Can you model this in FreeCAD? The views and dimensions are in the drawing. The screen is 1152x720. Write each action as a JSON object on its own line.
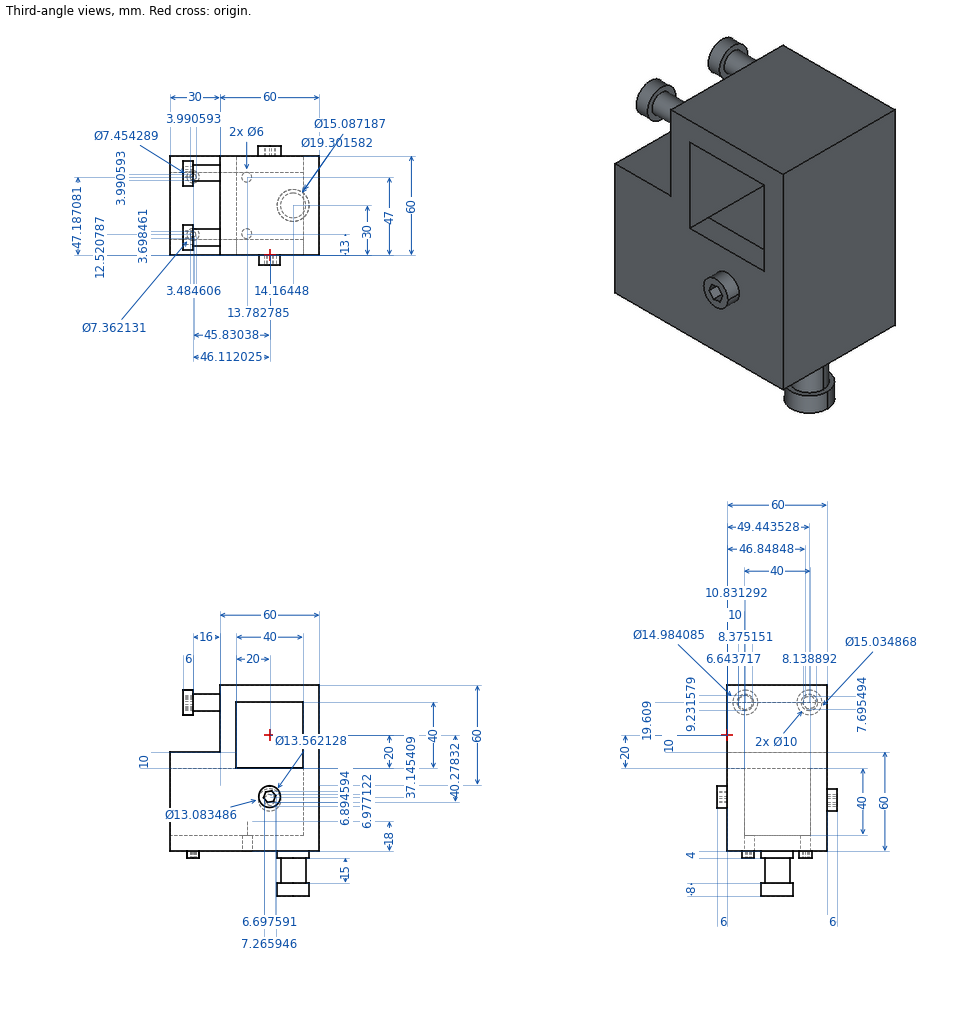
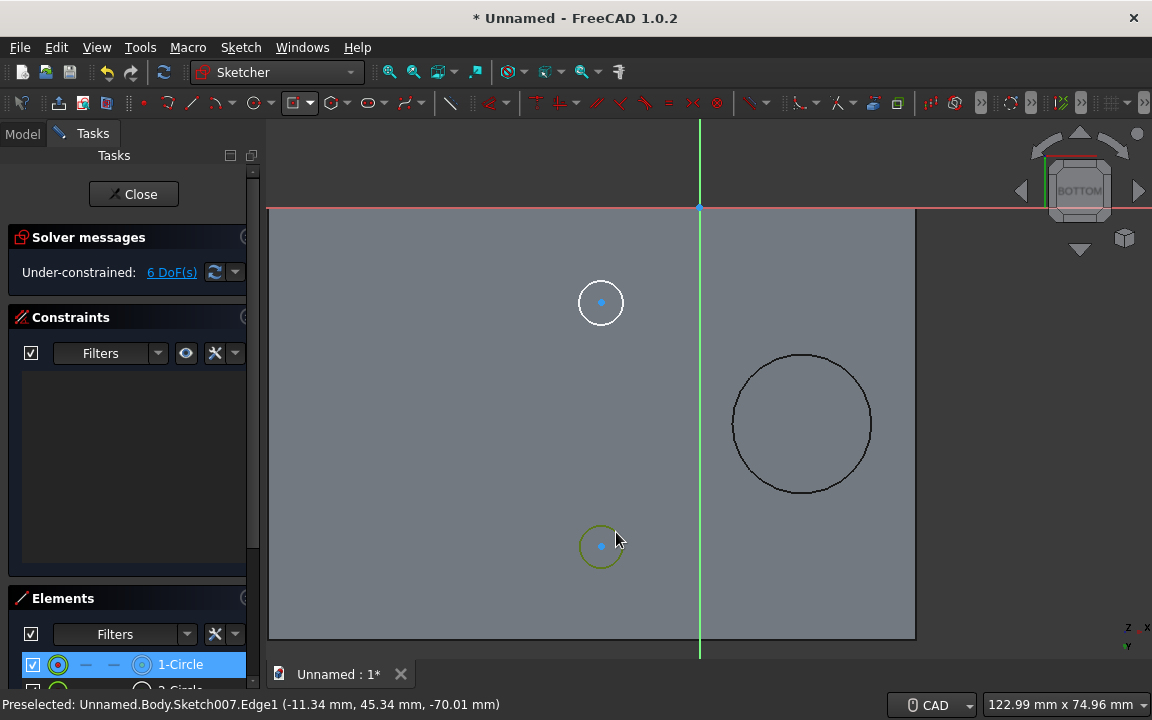
{"action": "left_click", "coordinate": [616, 287]}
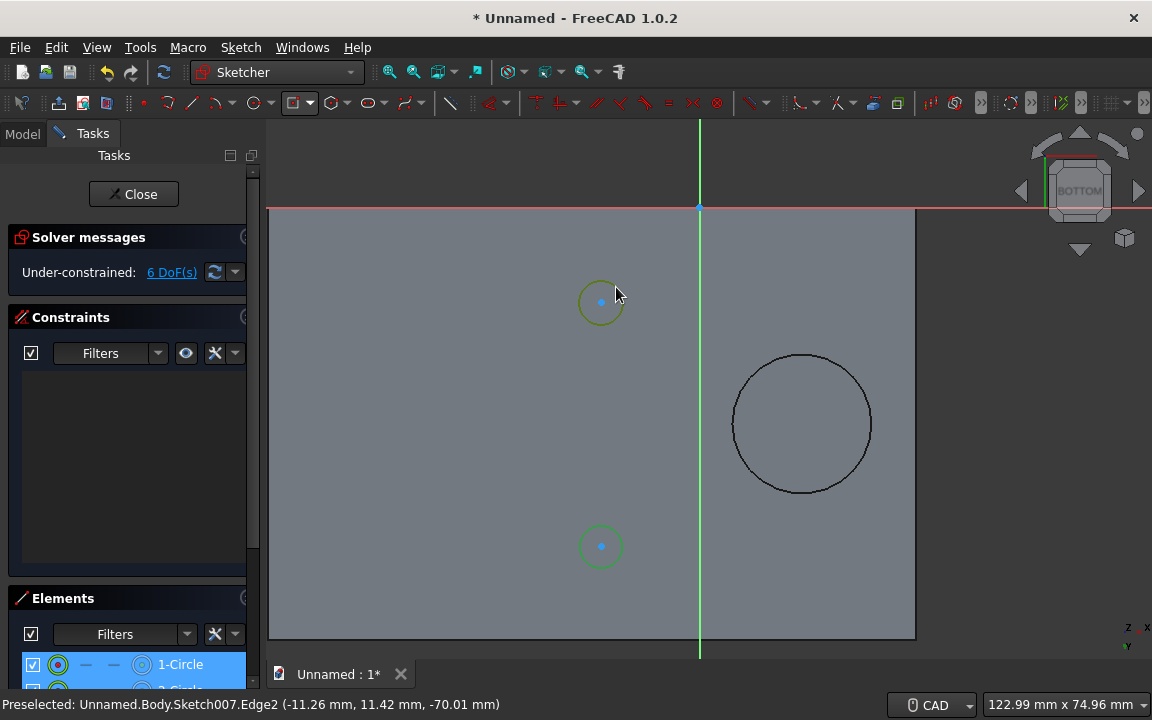
{"action": "left_click", "coordinate": [670, 104]}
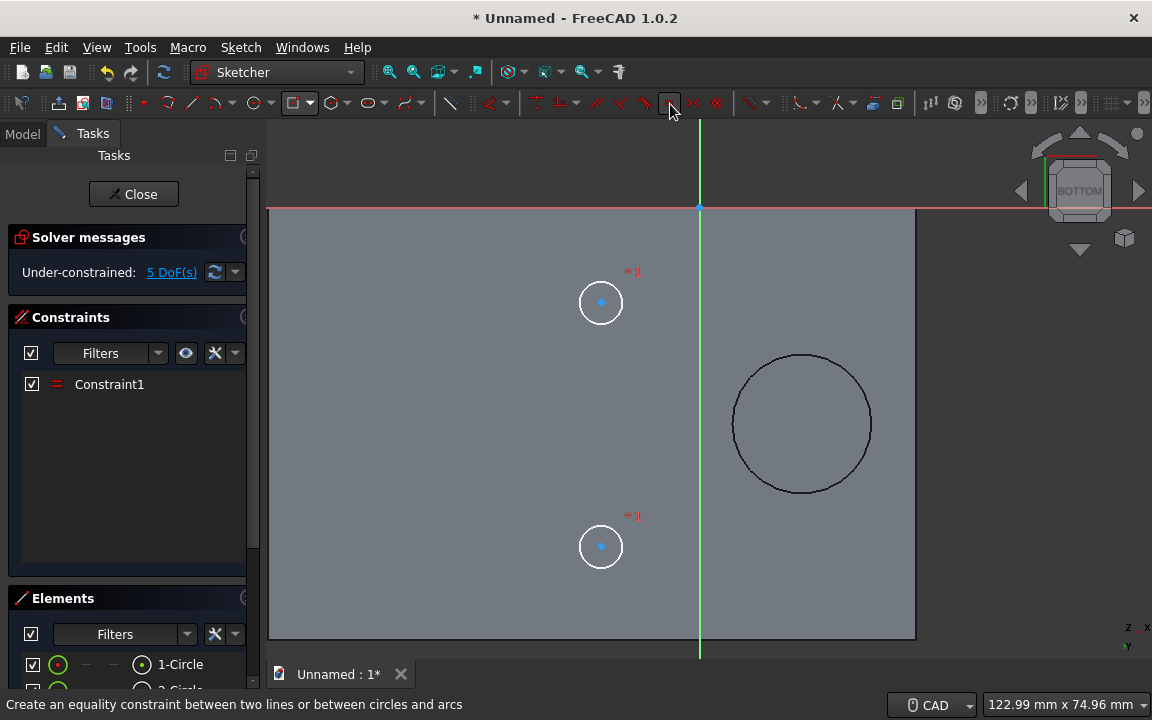
{"action": "left_click", "coordinate": [601, 547]}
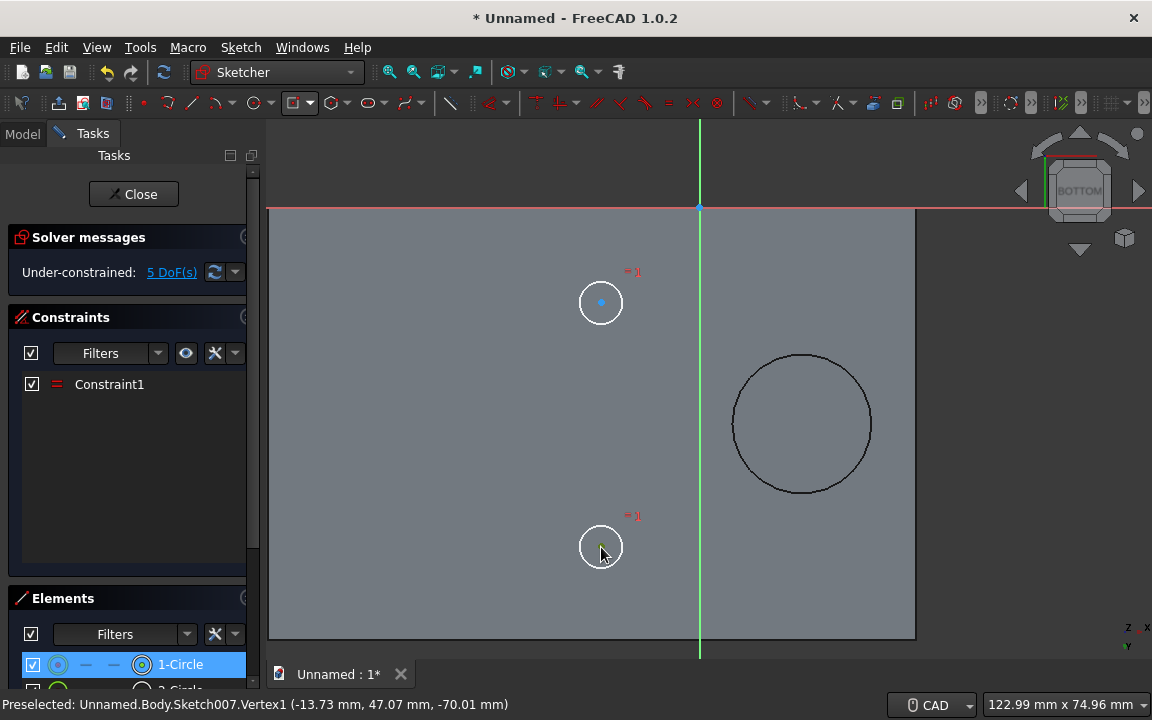
{"action": "left_click", "coordinate": [601, 303]}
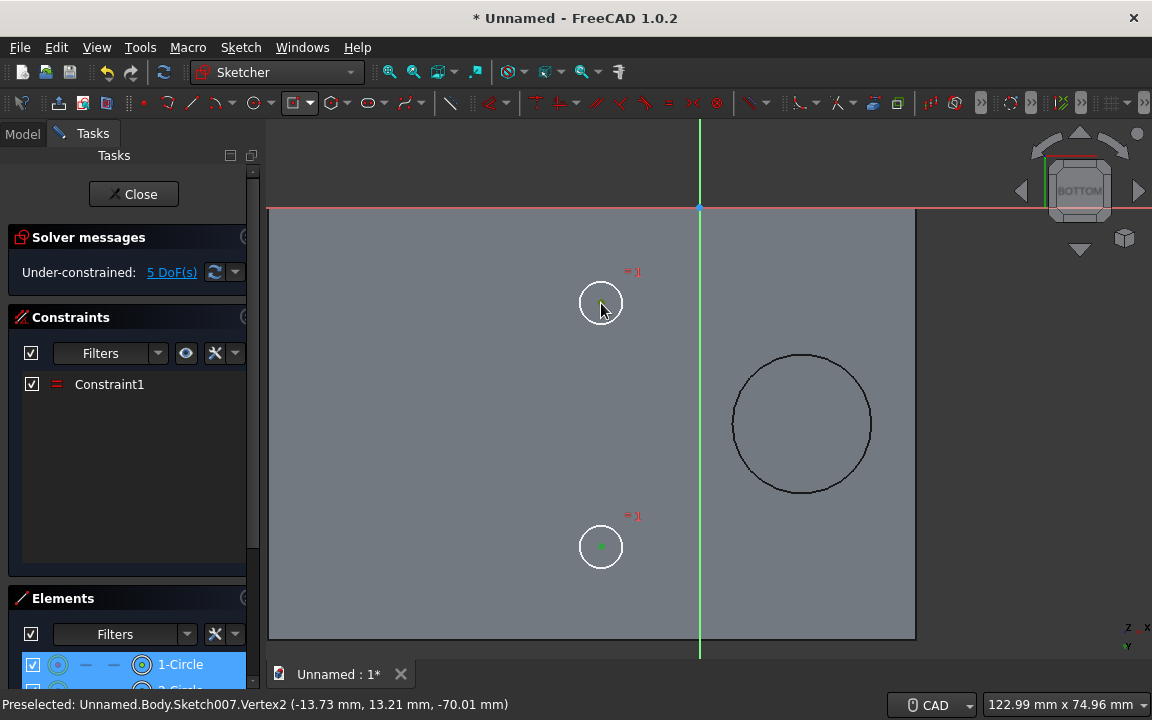
{"action": "left_click", "coordinate": [578, 104]}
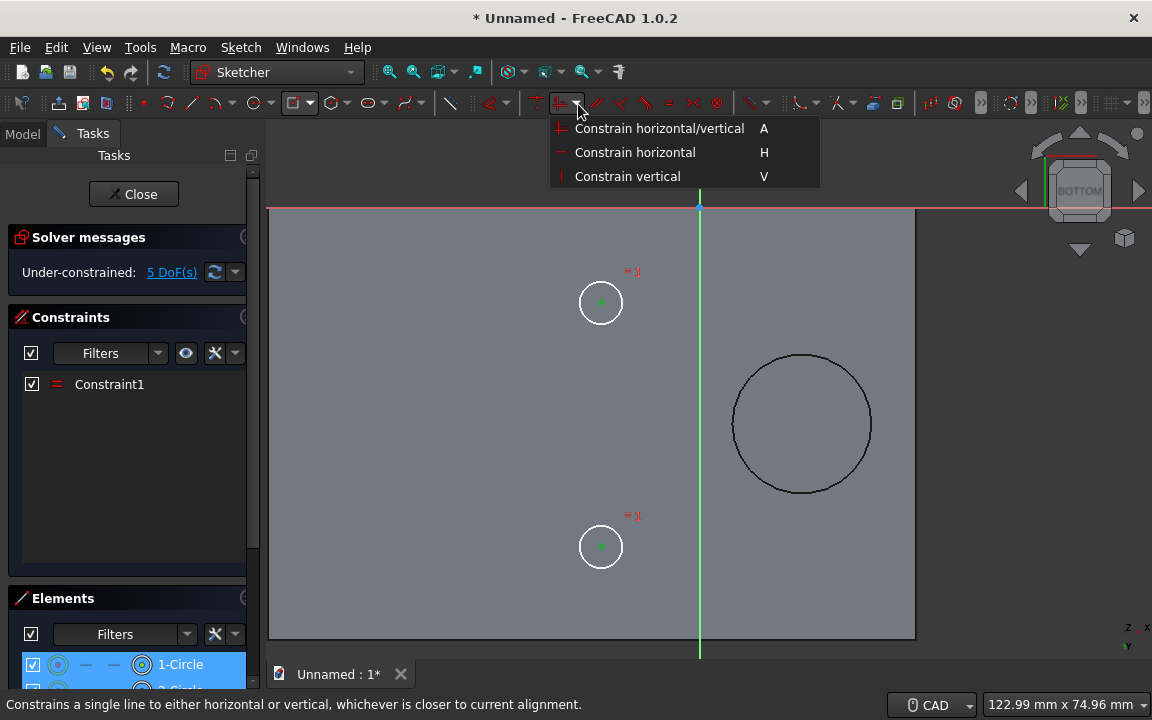
{"action": "left_click", "coordinate": [685, 176]}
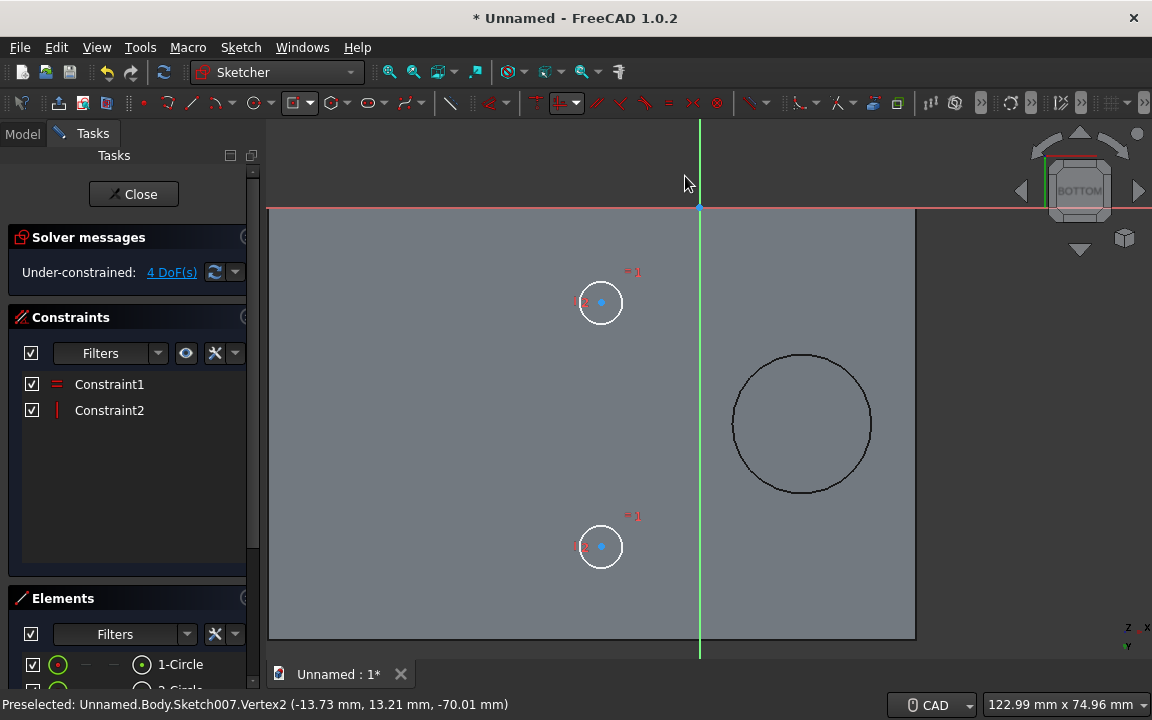
{"action": "left_click", "coordinate": [490, 104]}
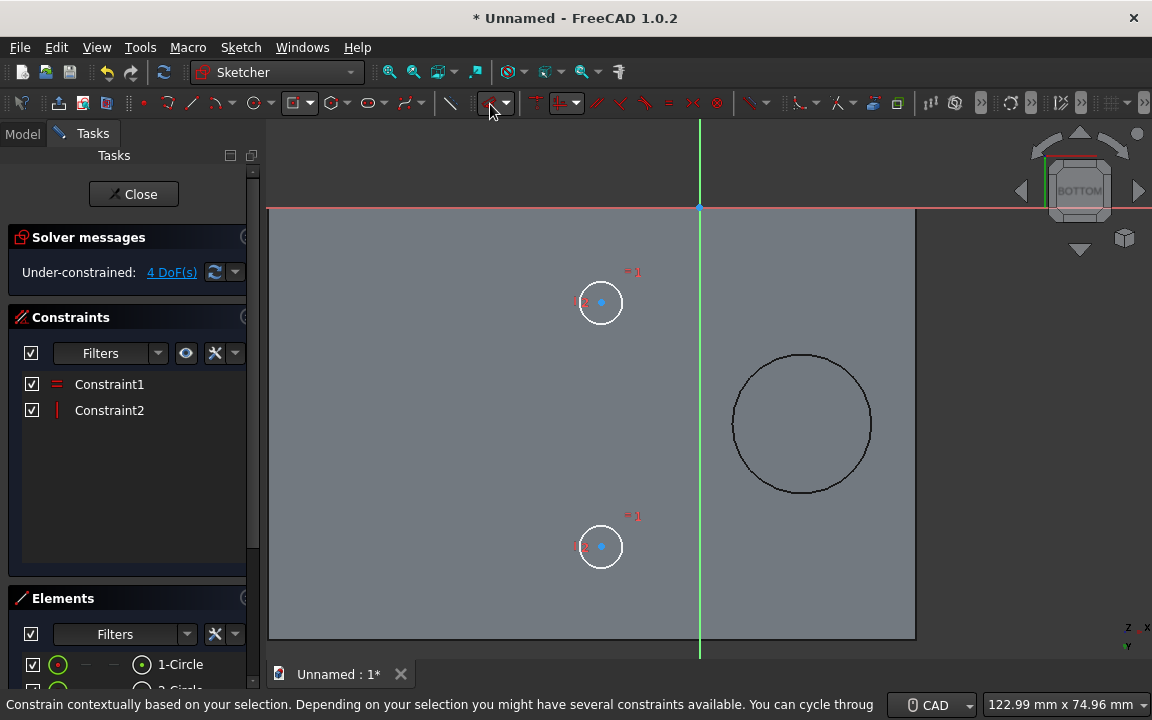
{"action": "left_click", "coordinate": [616, 532]}
{"action": "left_click", "coordinate": [639, 509]}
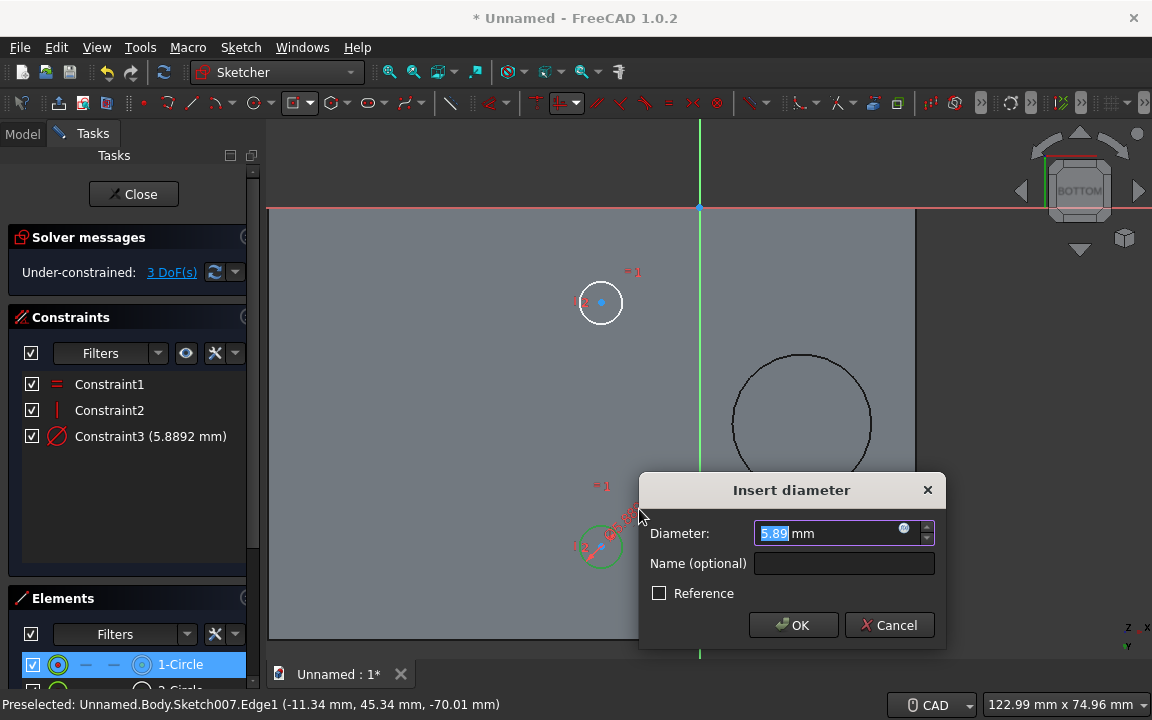
{"action": "type", "text": "6"}
{"action": "key", "text": "Return"}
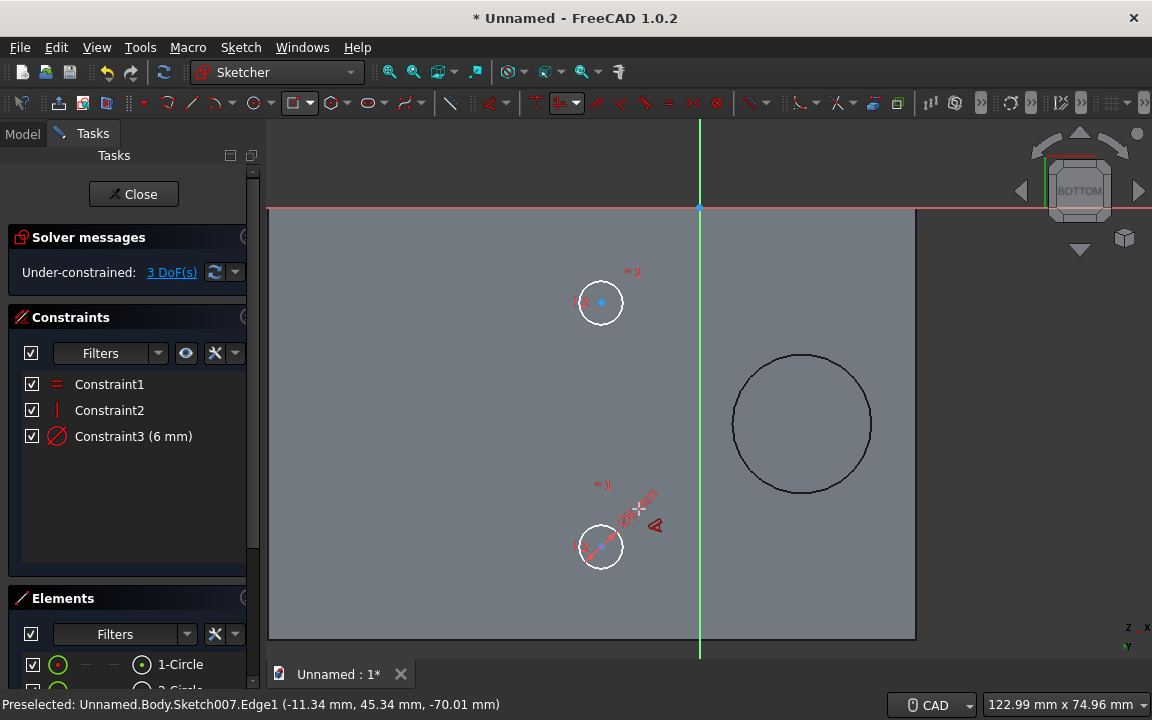
{"action": "left_click", "coordinate": [601, 547]}
{"action": "left_click", "coordinate": [734, 377]}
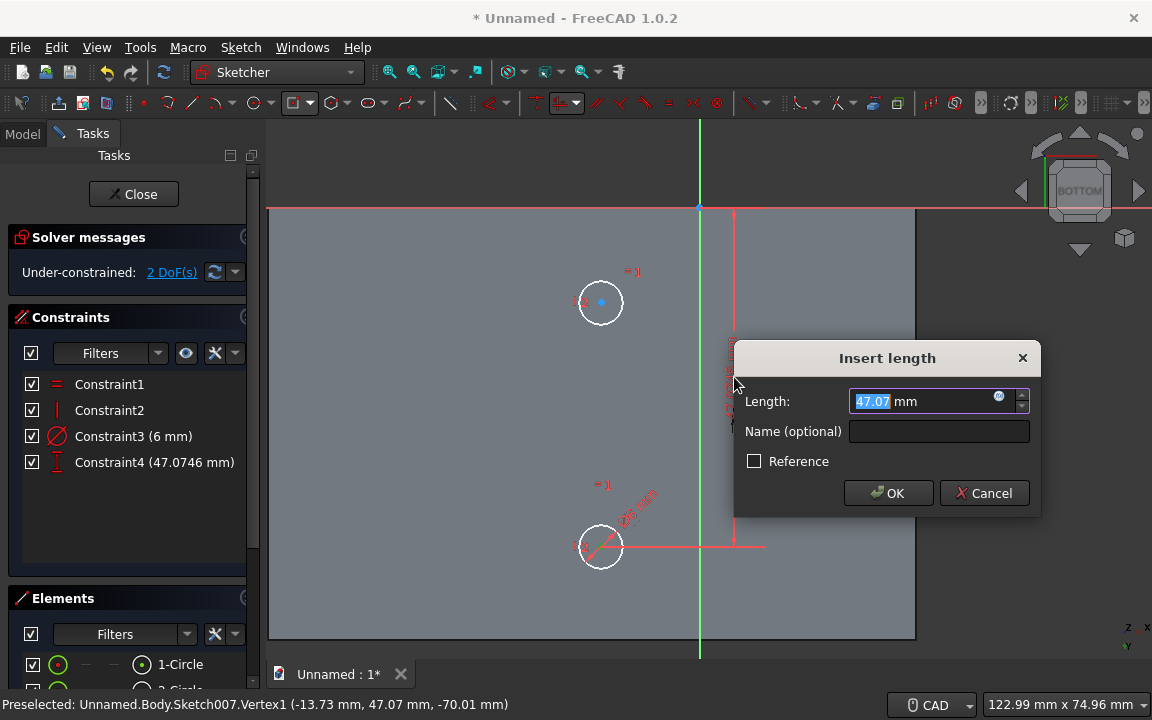
{"action": "type", "text": "47"}
{"action": "key", "text": "Return"}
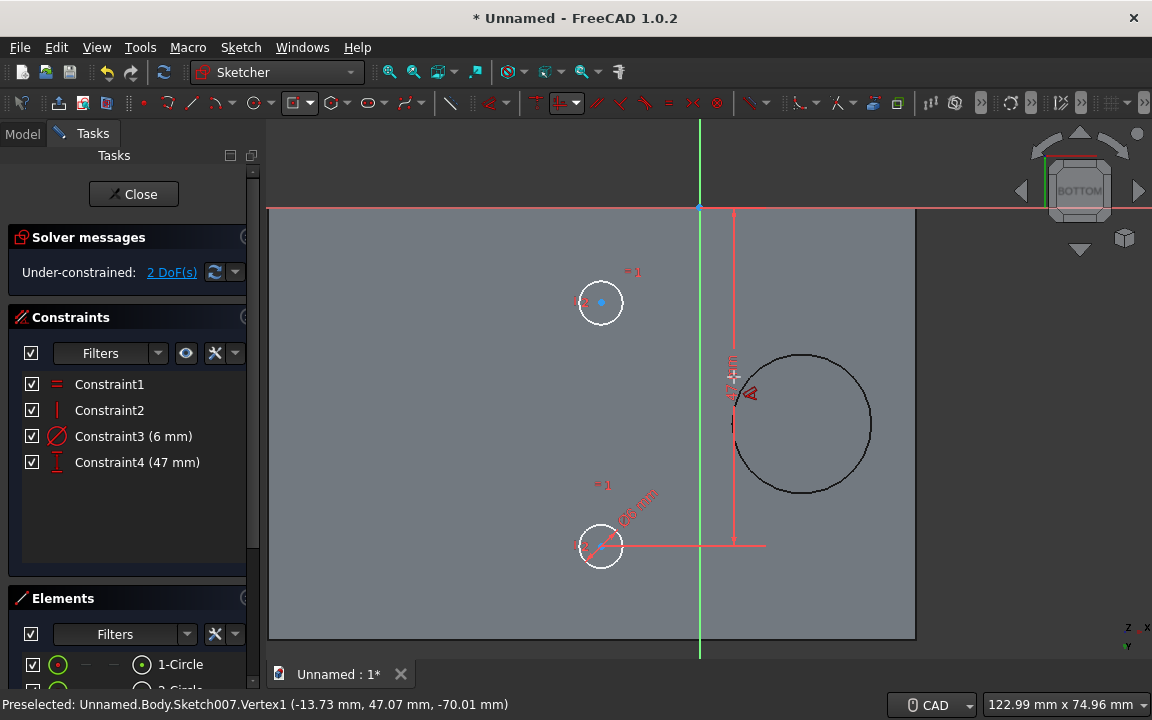
{"action": "left_click", "coordinate": [601, 303]}
{"action": "left_click", "coordinate": [734, 255]}